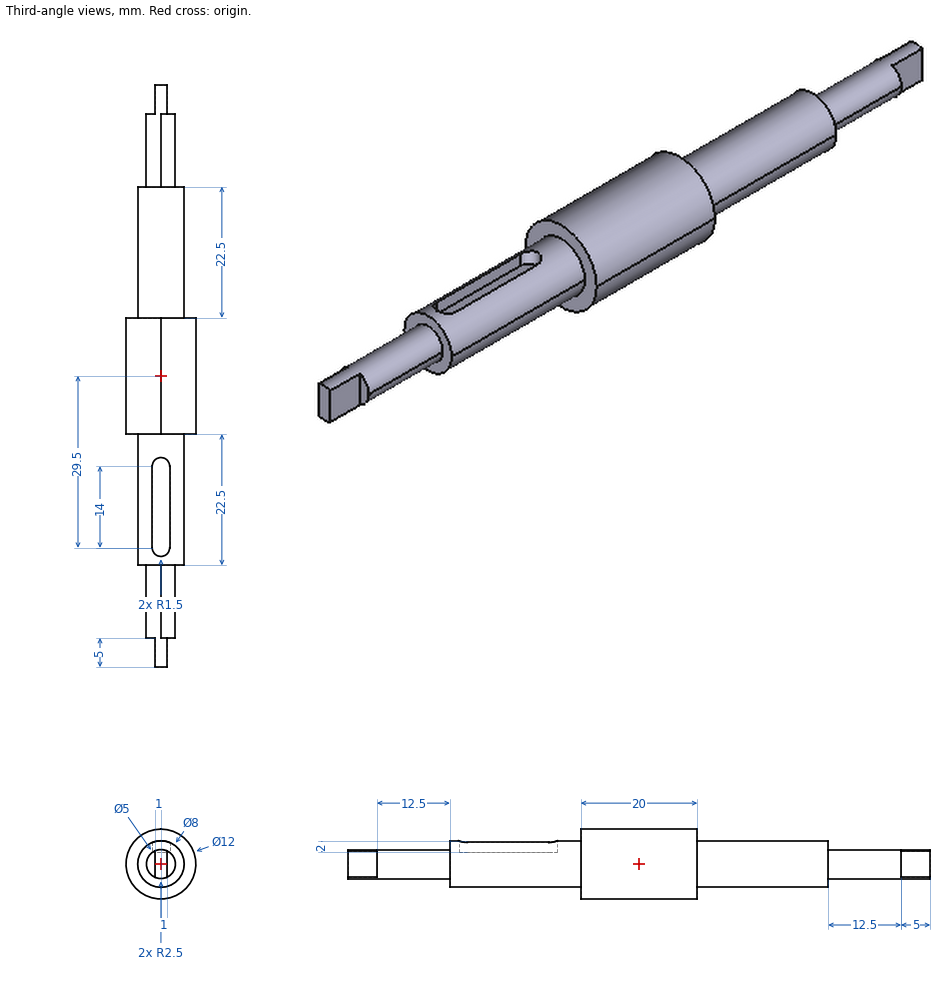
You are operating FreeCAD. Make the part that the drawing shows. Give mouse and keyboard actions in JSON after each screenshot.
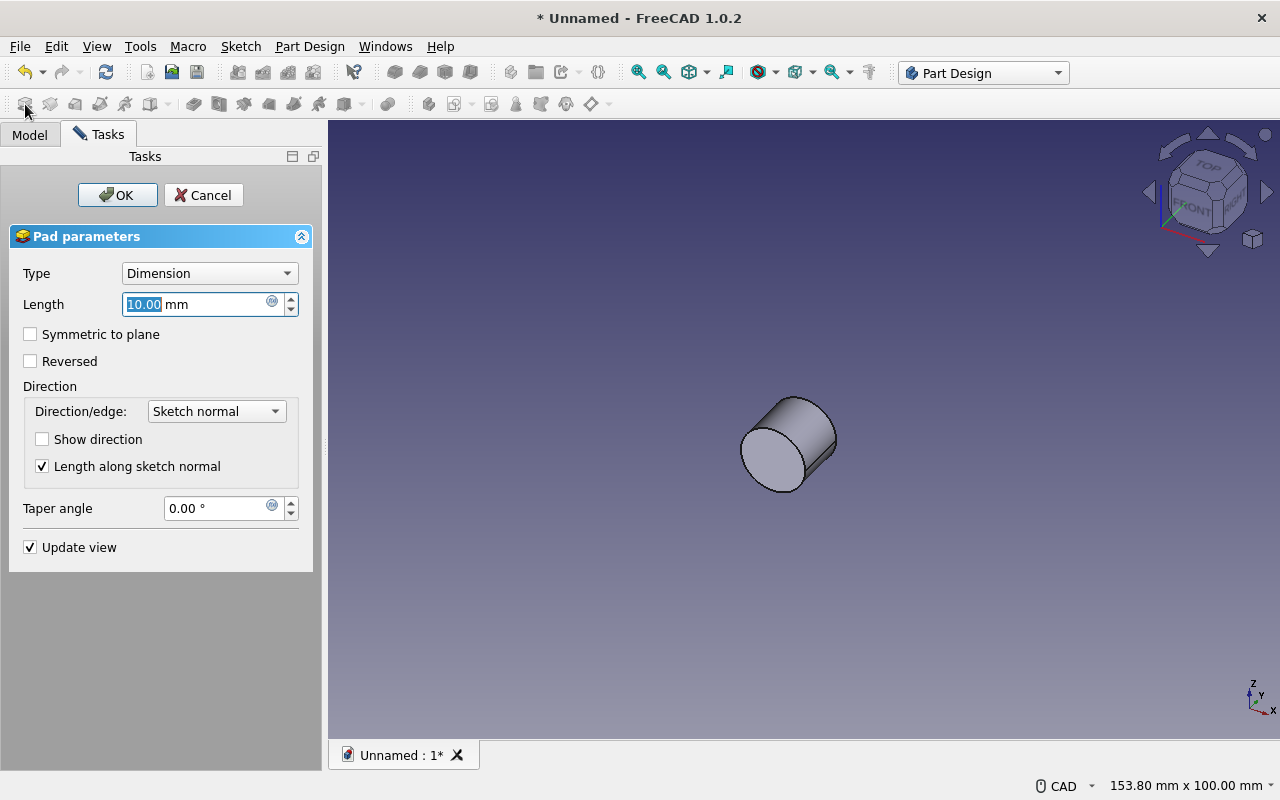
{"action": "type", "text": "20"}
{"action": "key", "text": "Tab"}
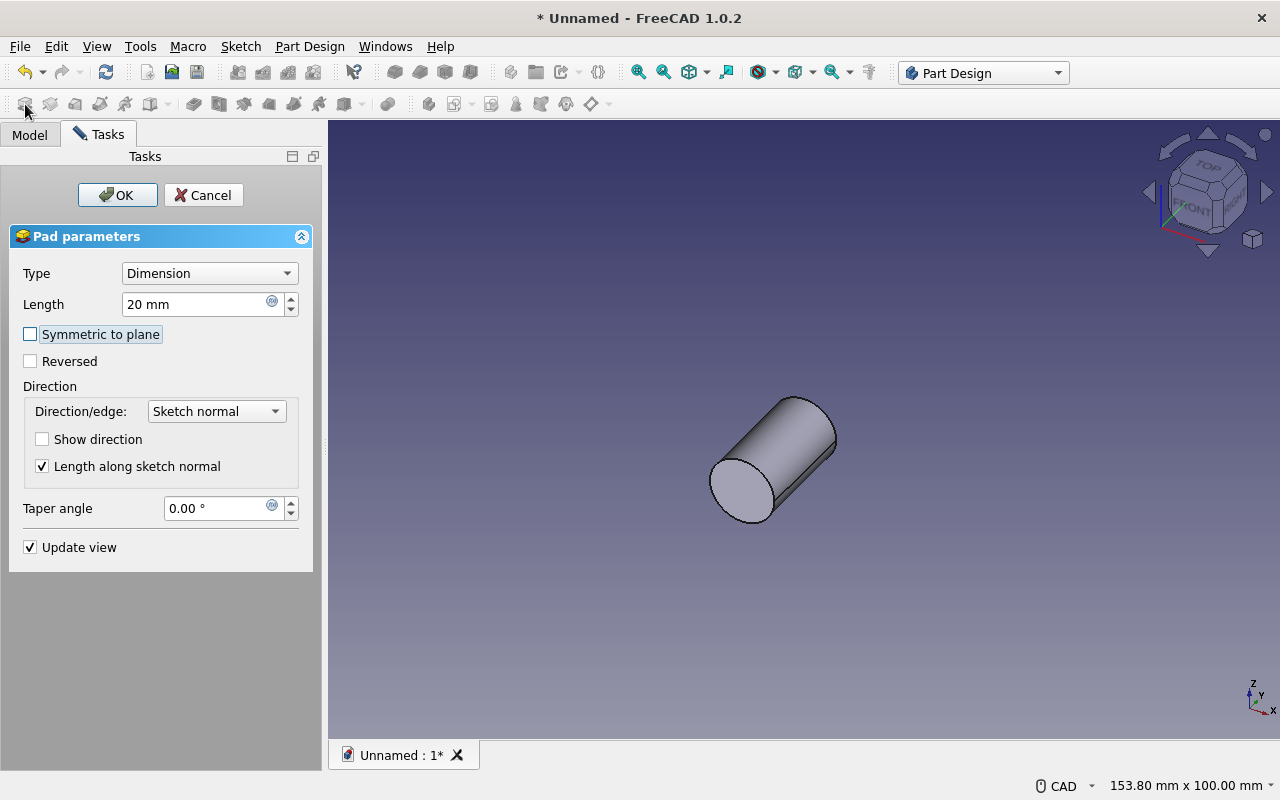
{"action": "left_click", "coordinate": [31, 334]}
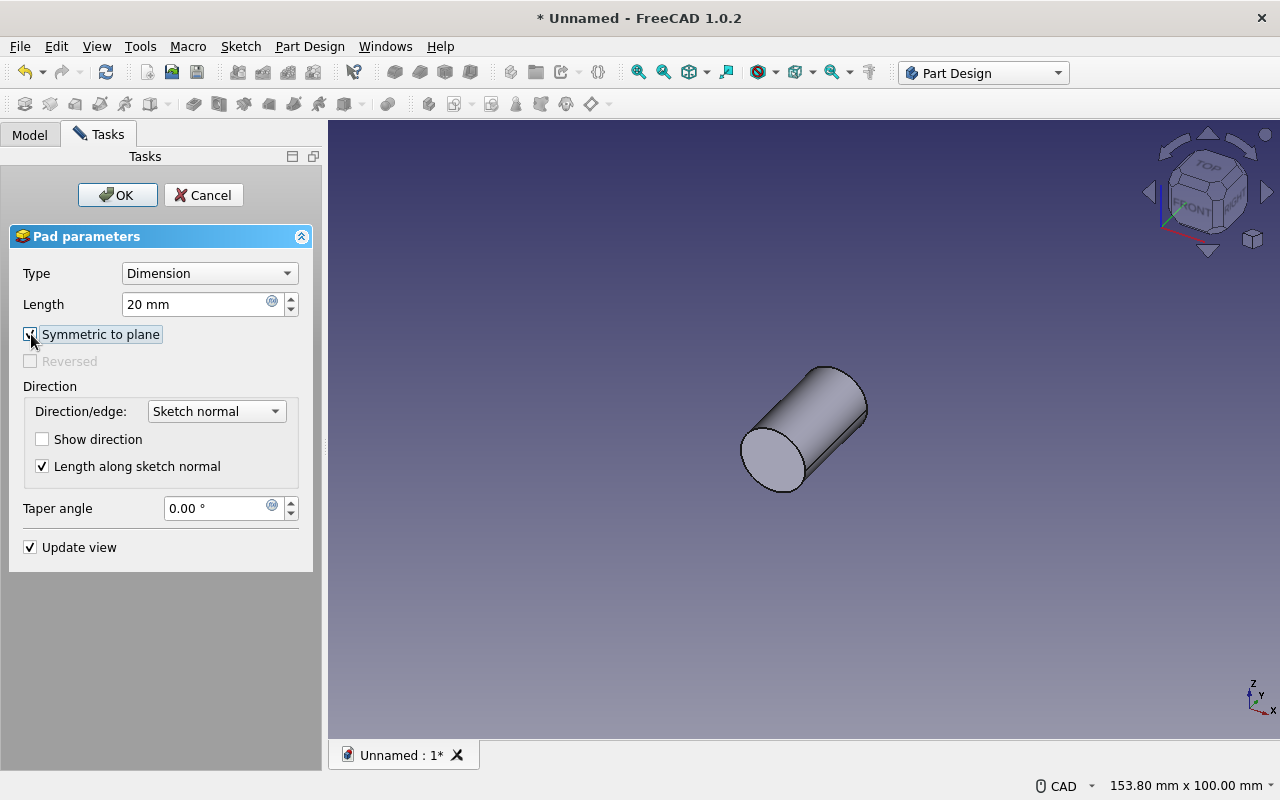
{"action": "left_click", "coordinate": [118, 195]}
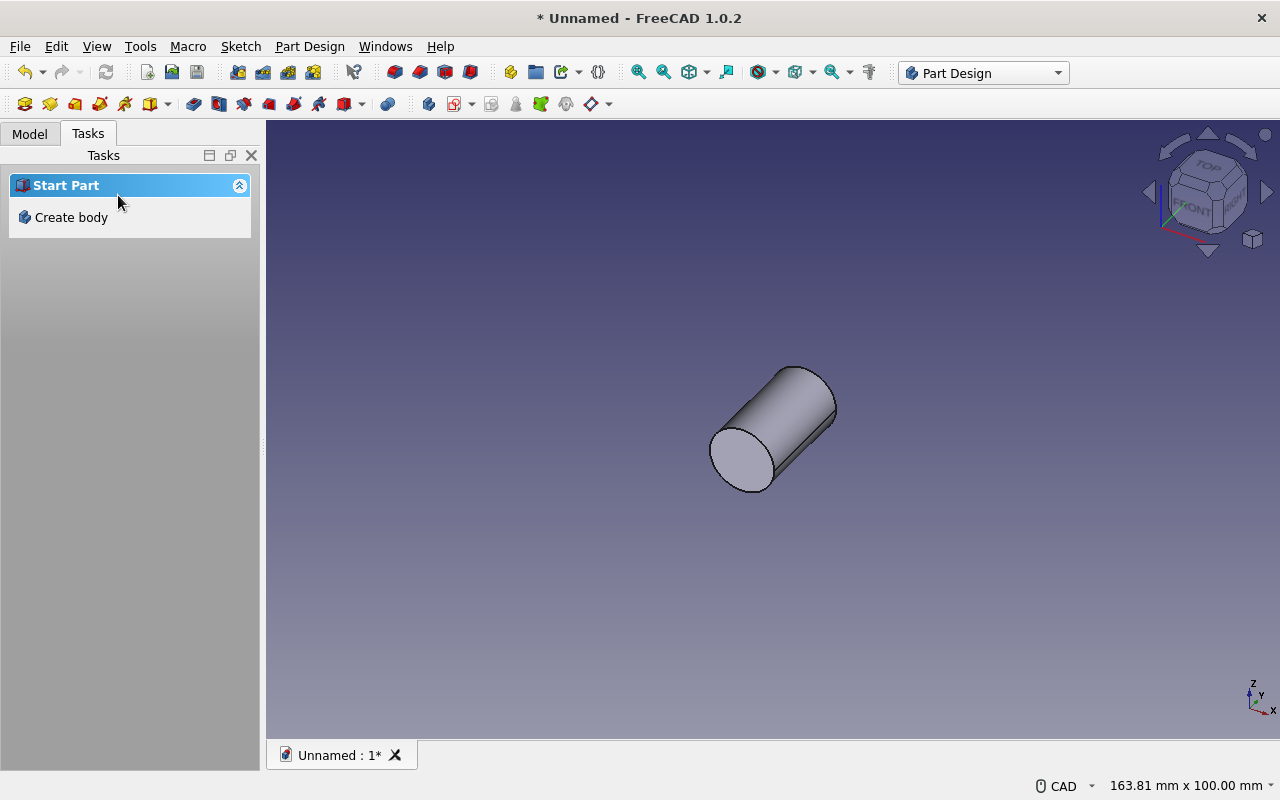
{"action": "key", "text": "v f"}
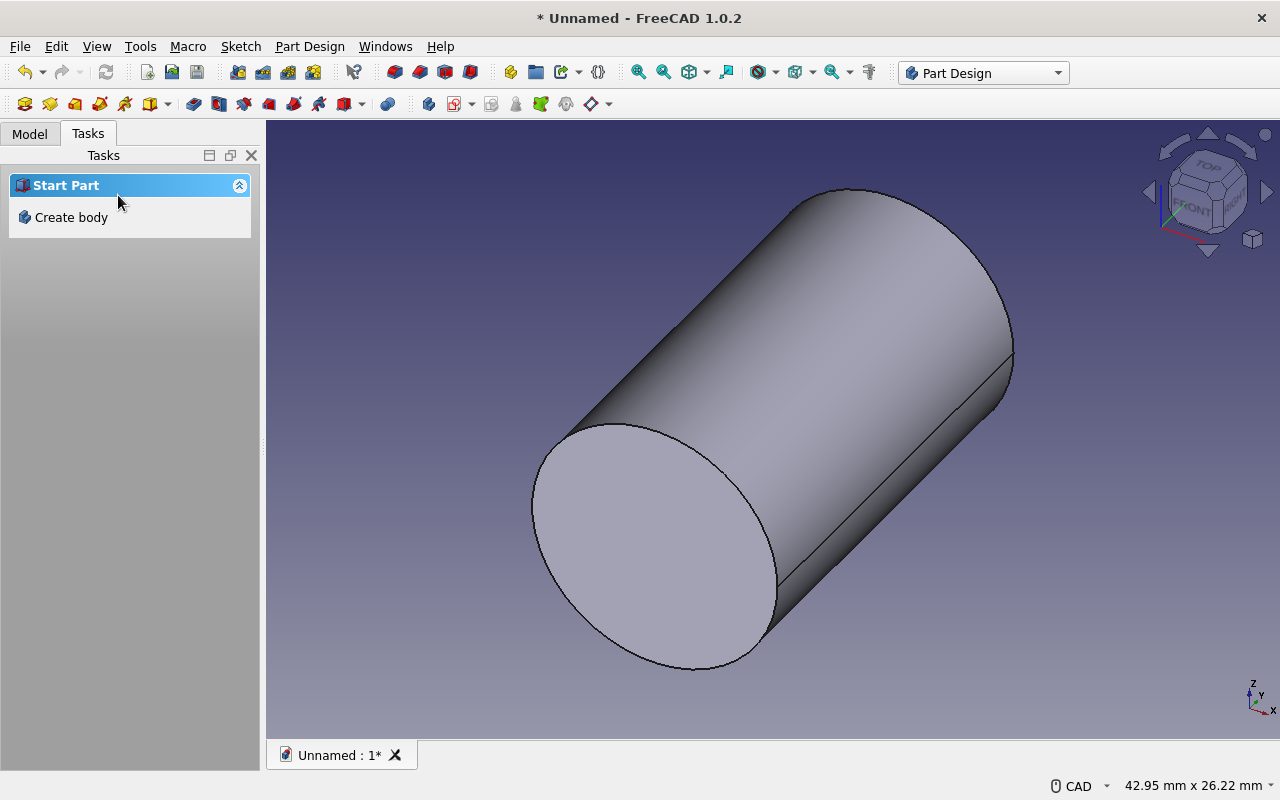
{"action": "key", "text": "4"}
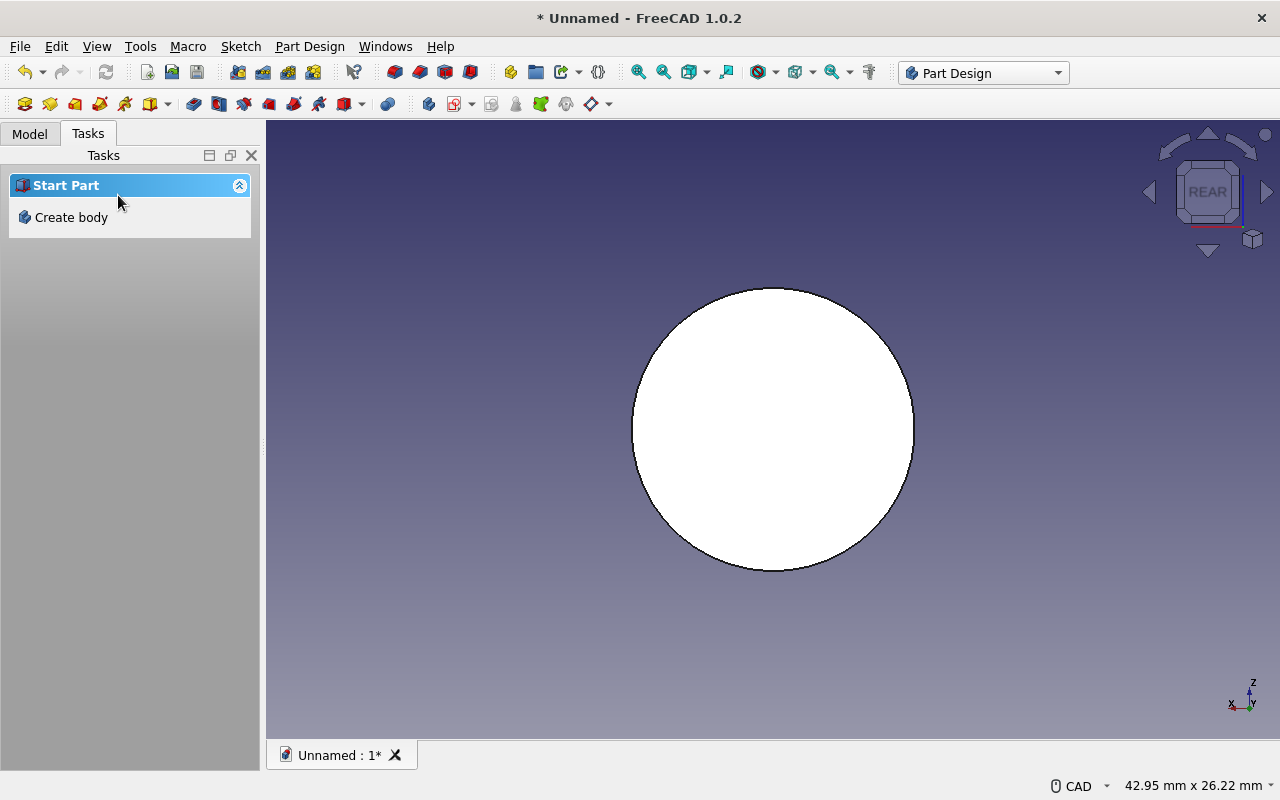
{"action": "left_click", "coordinate": [773, 428]}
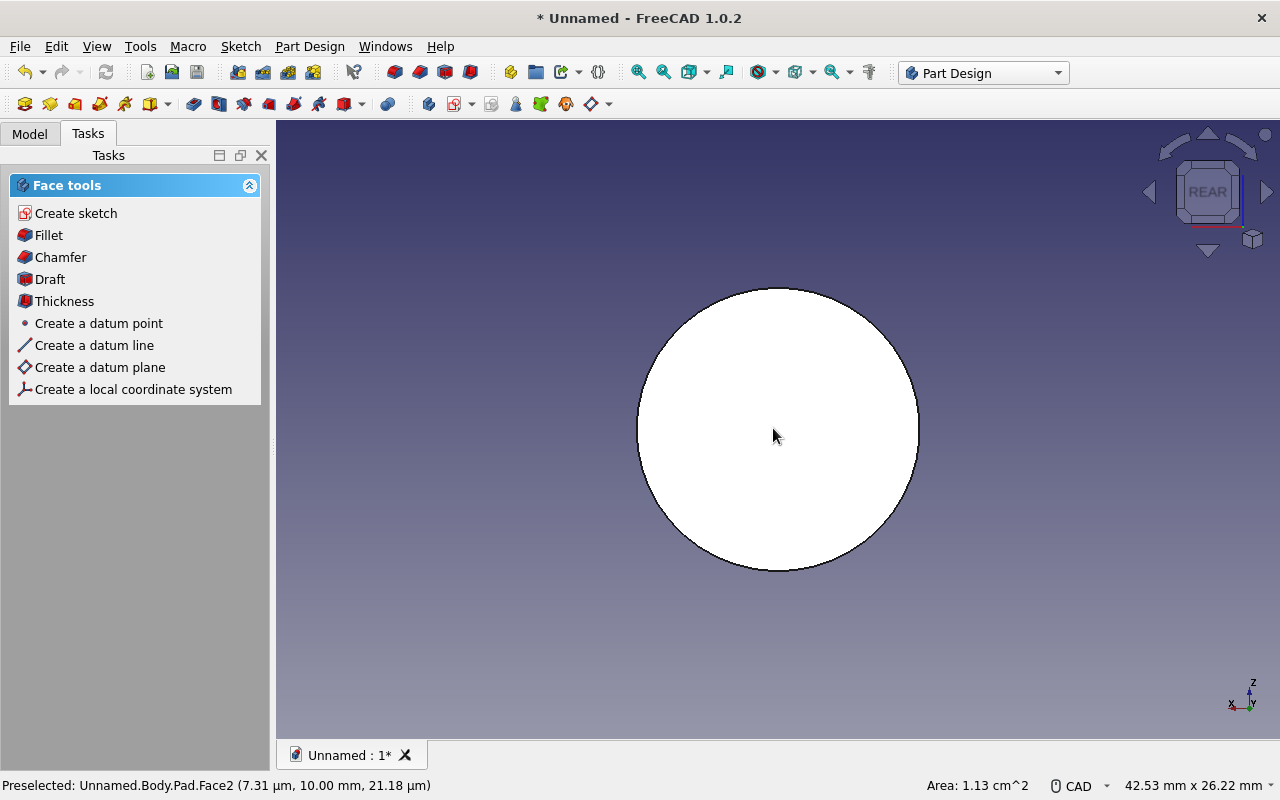
{"action": "left_click", "coordinate": [454, 104]}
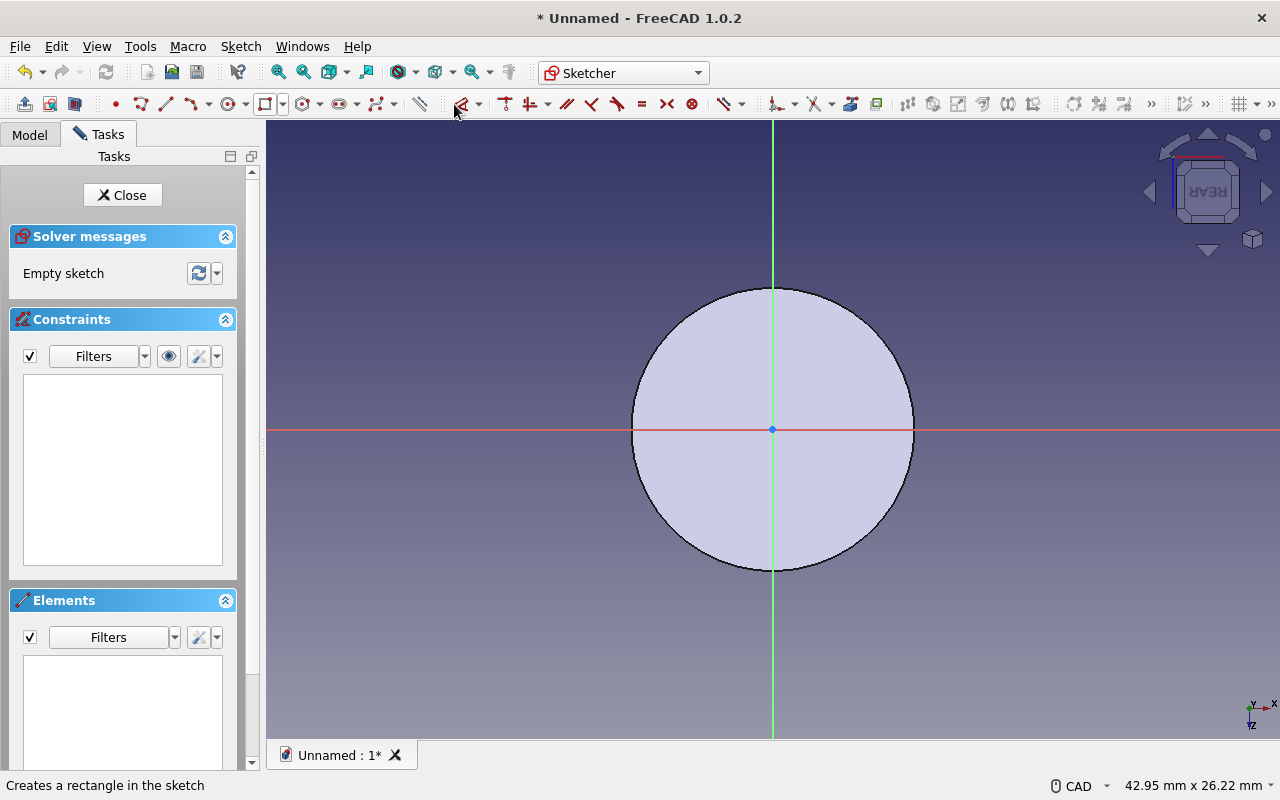
{"action": "scroll", "coordinate": [829, 430], "scroll_direction": "up", "scroll_amount": 4}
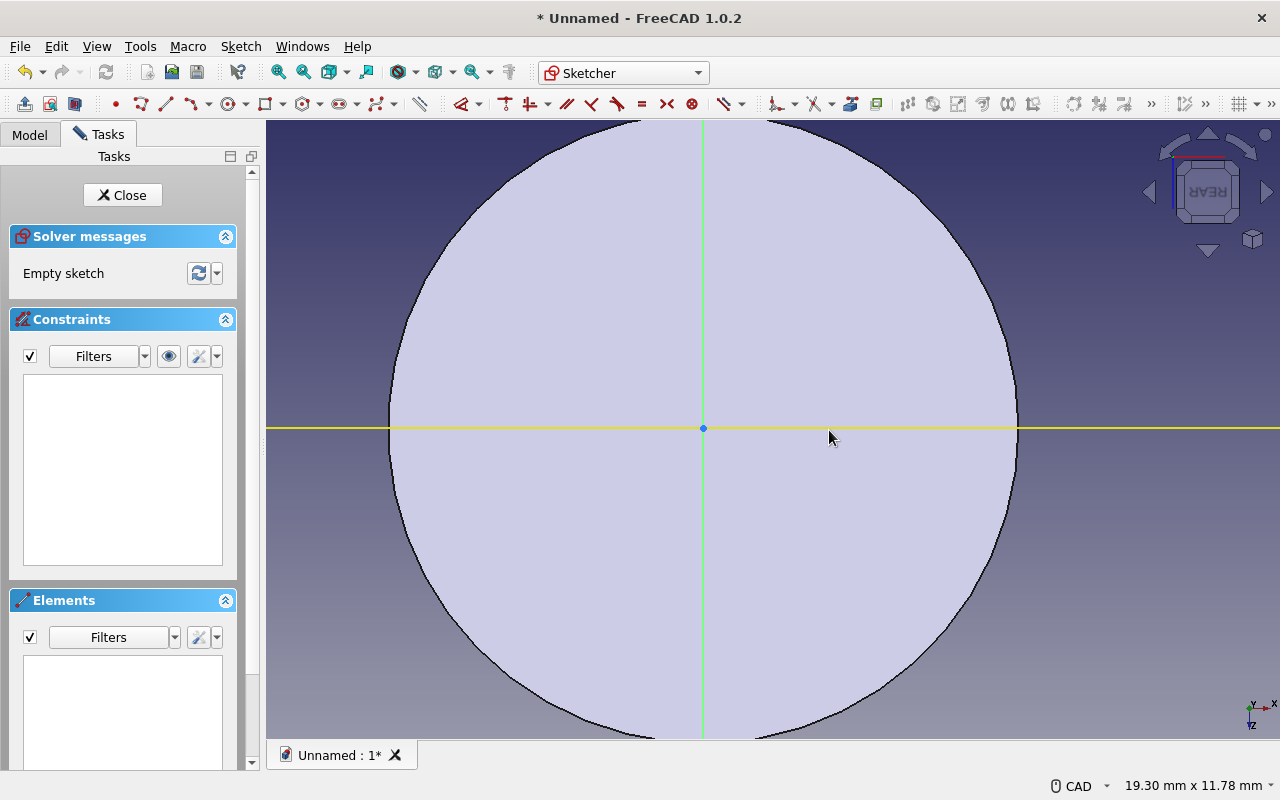
{"action": "key", "text": "g c"}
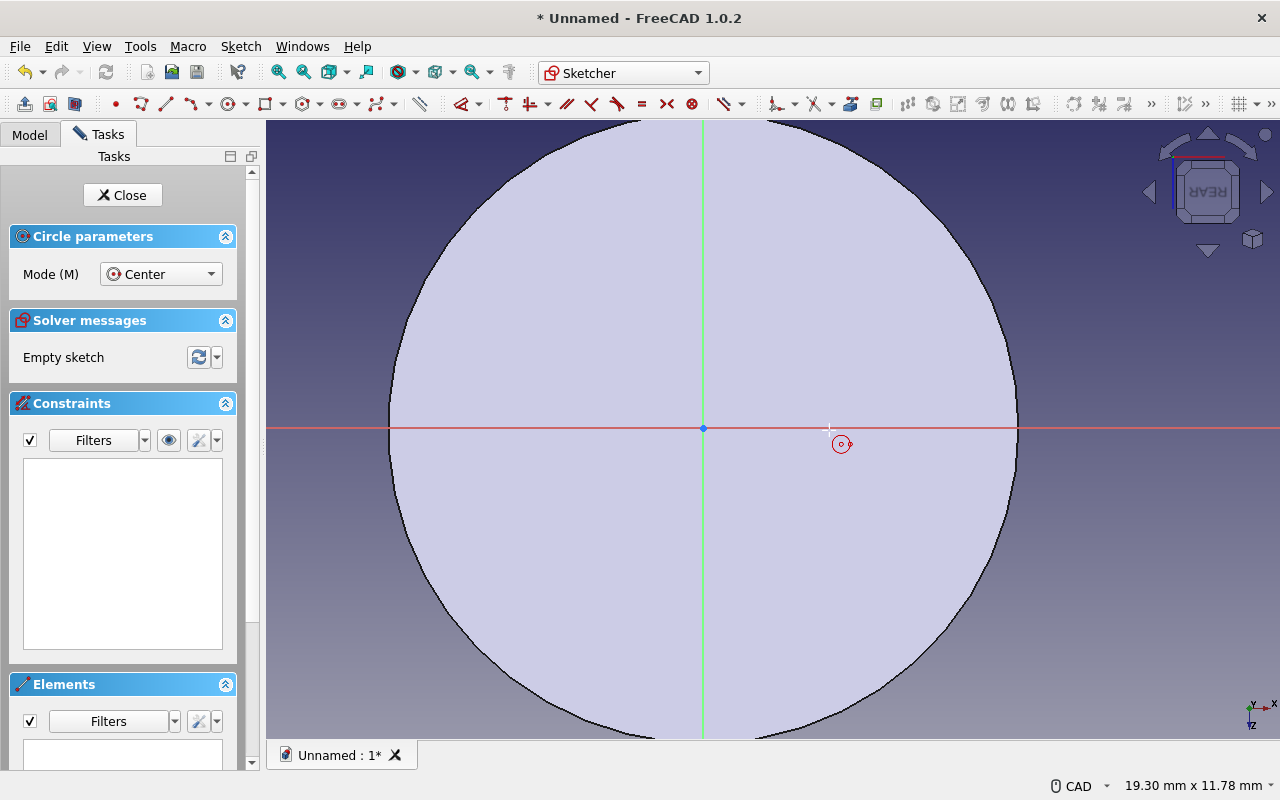
{"action": "left_click", "coordinate": [703, 428]}
{"action": "mouse_move", "coordinate": [852, 280]}